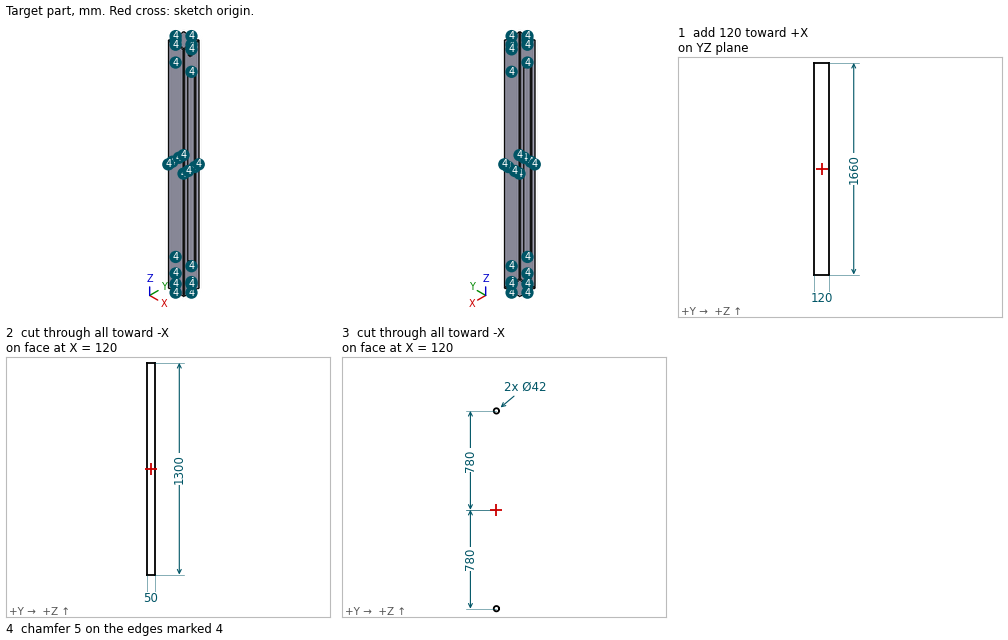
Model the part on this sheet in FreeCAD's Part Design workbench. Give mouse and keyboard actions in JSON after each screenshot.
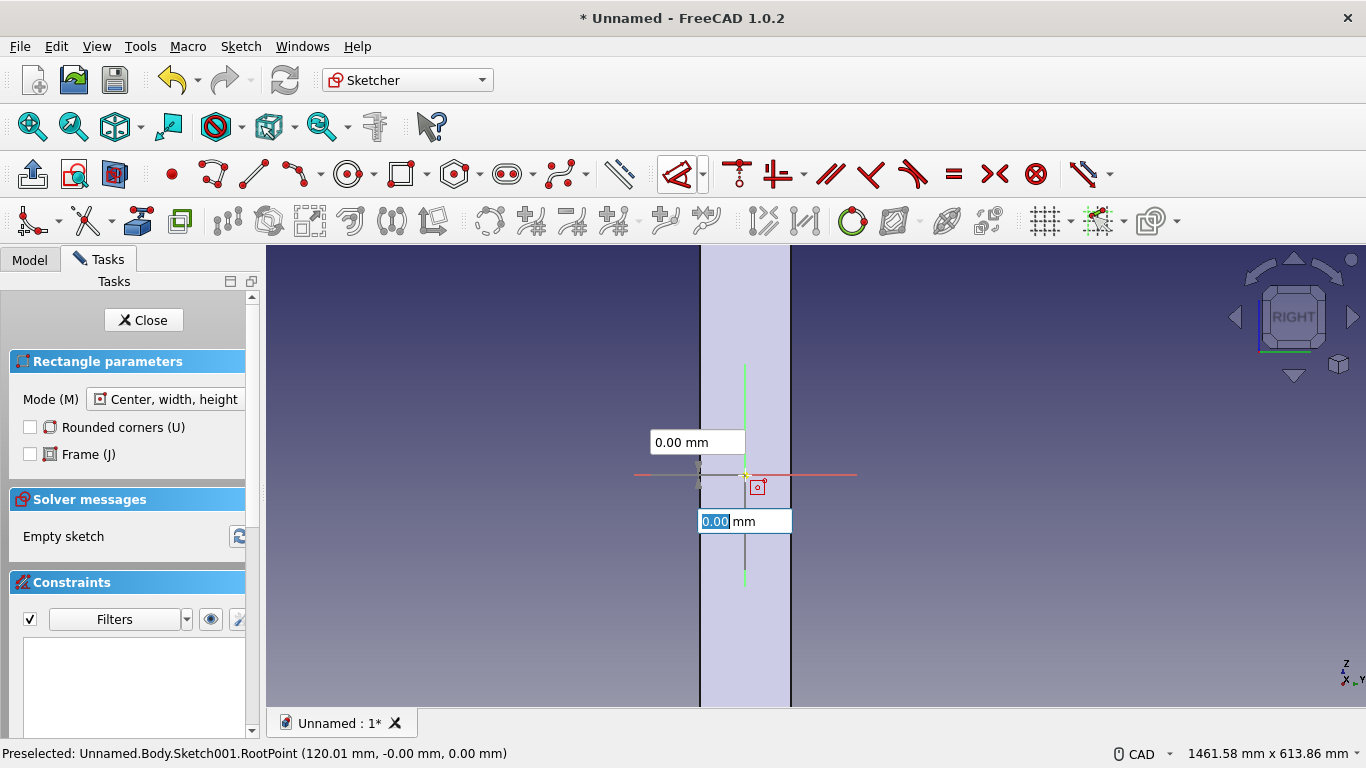
{"action": "scroll", "coordinate": [748, 476], "scroll_direction": "down", "scroll_amount": 6}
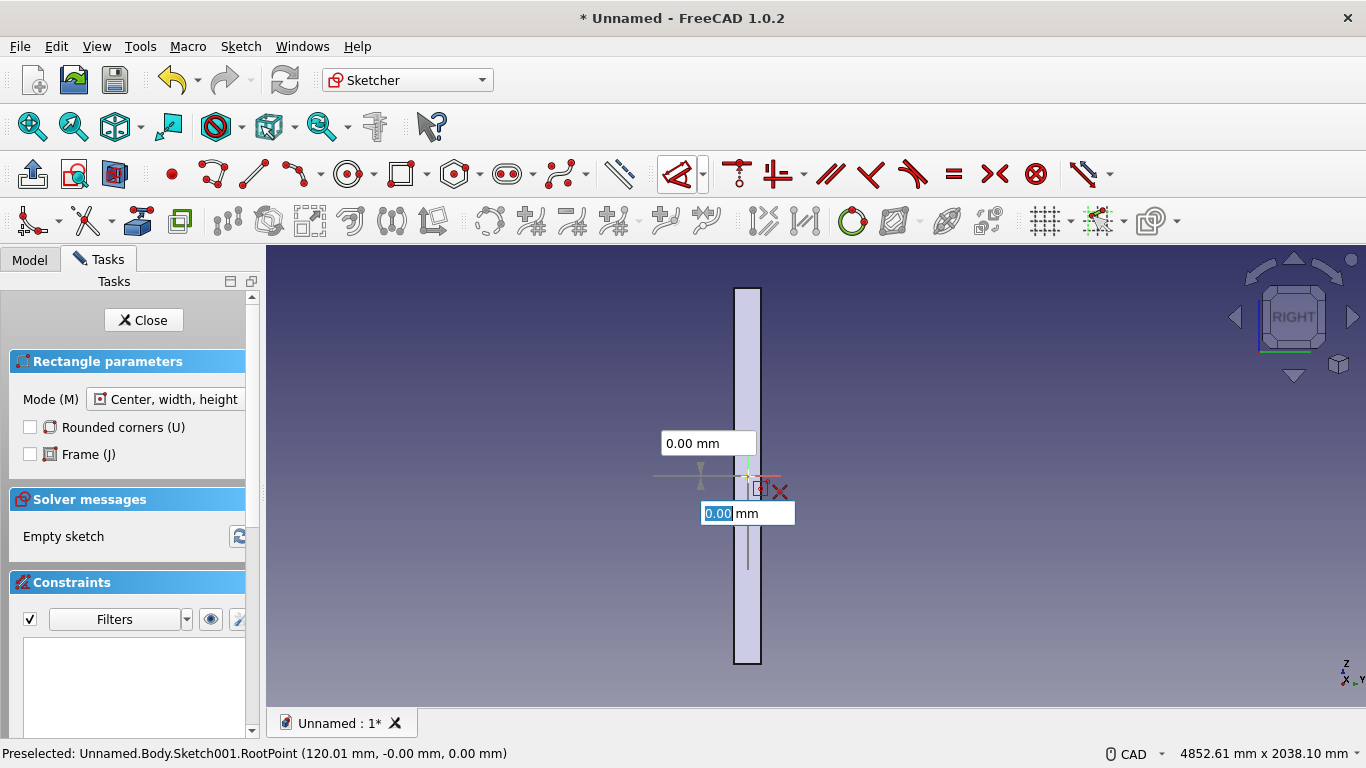
{"action": "scroll", "coordinate": [753, 329], "scroll_direction": "up", "scroll_amount": 6}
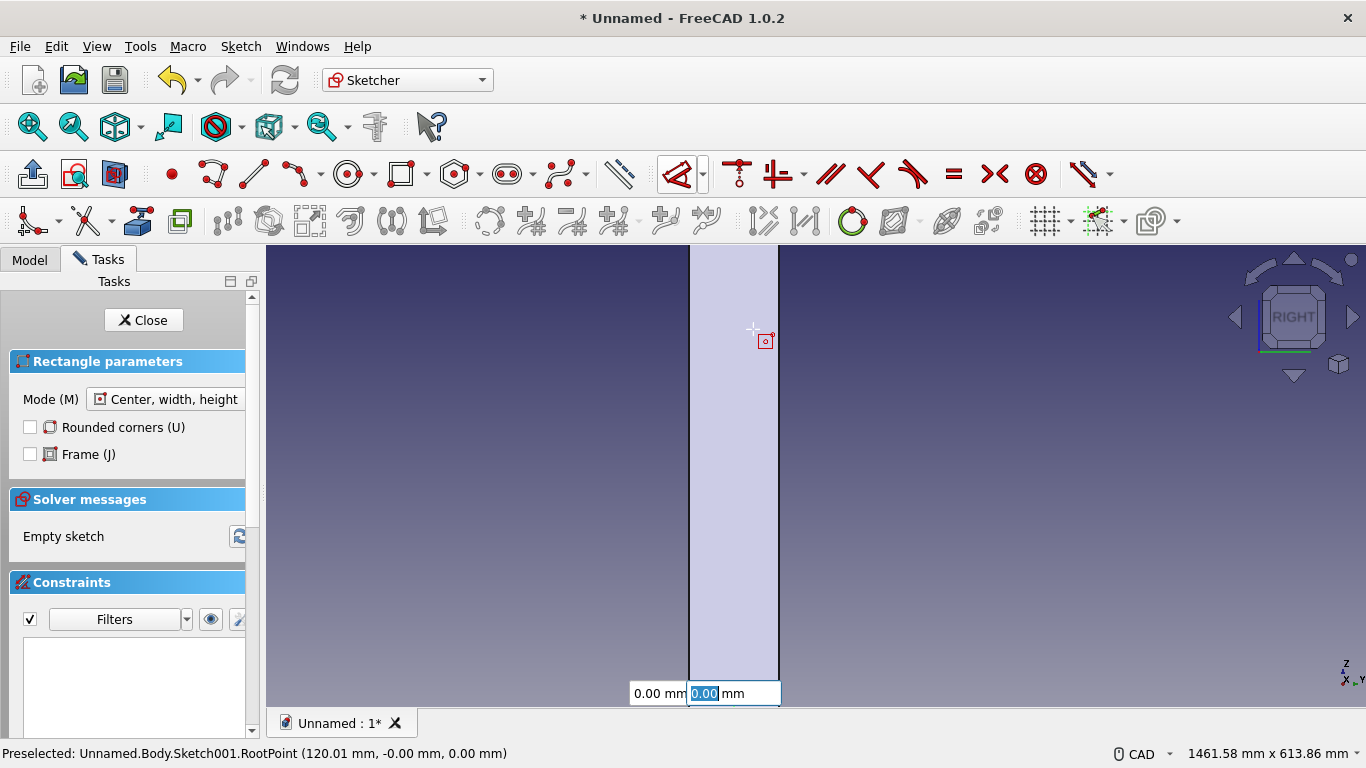
{"action": "left_click", "coordinate": [753, 328]}
{"action": "key", "text": "Escape"}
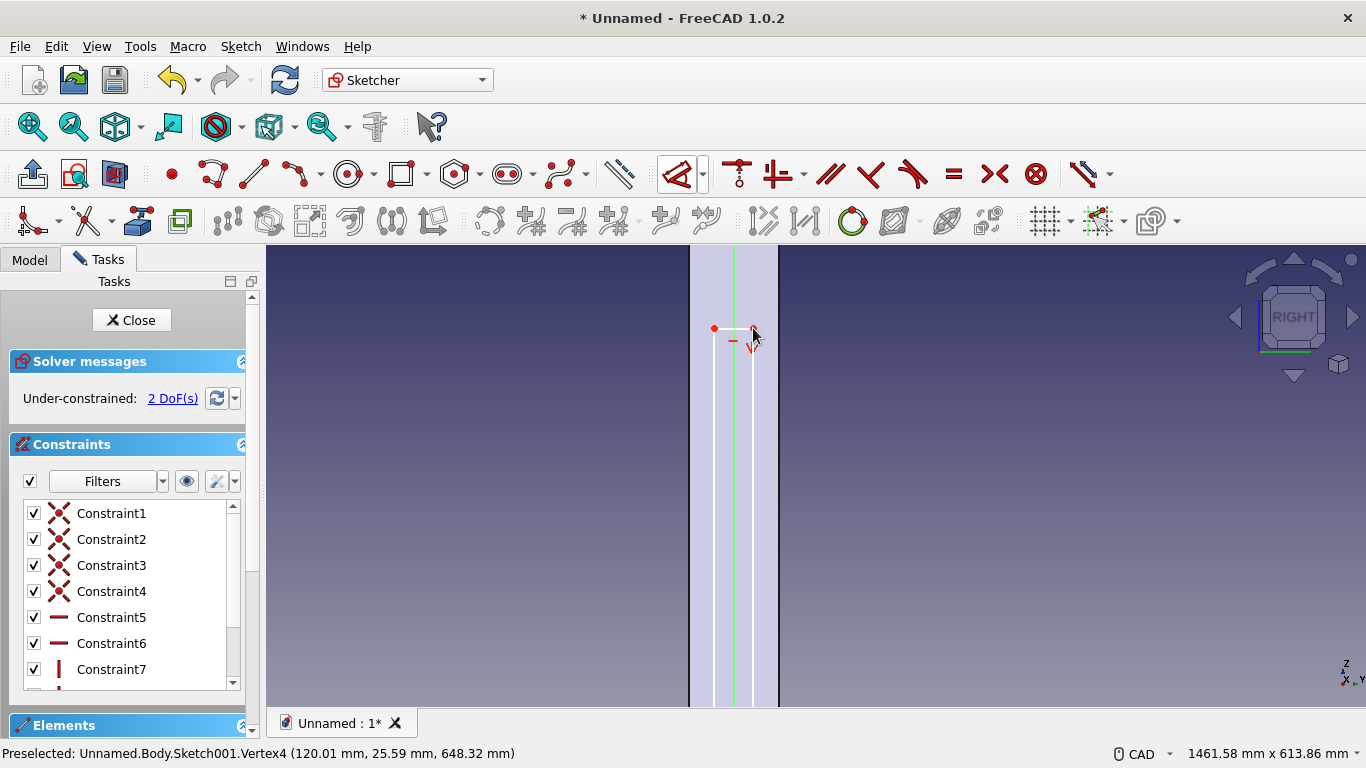
{"action": "key", "text": "d"}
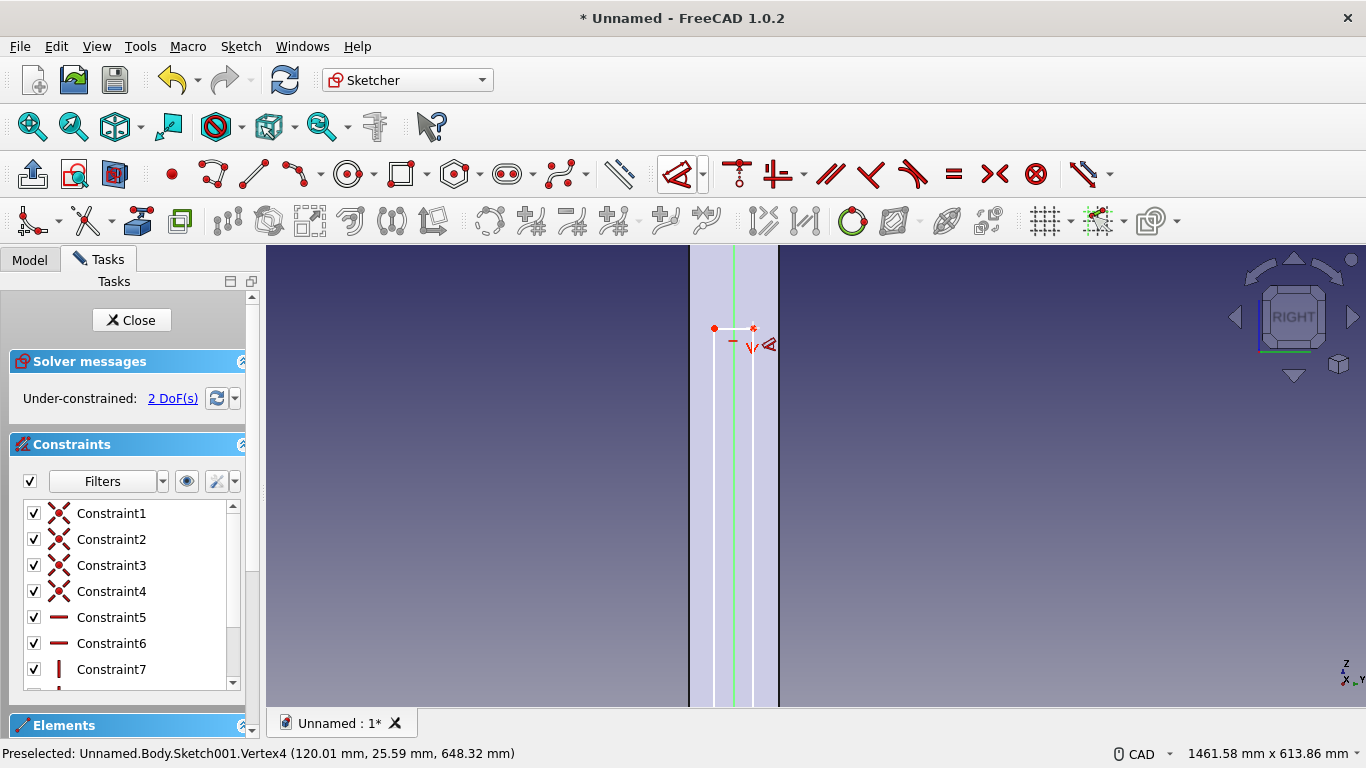
{"action": "scroll", "coordinate": [753, 329], "scroll_direction": "down", "scroll_amount": 6}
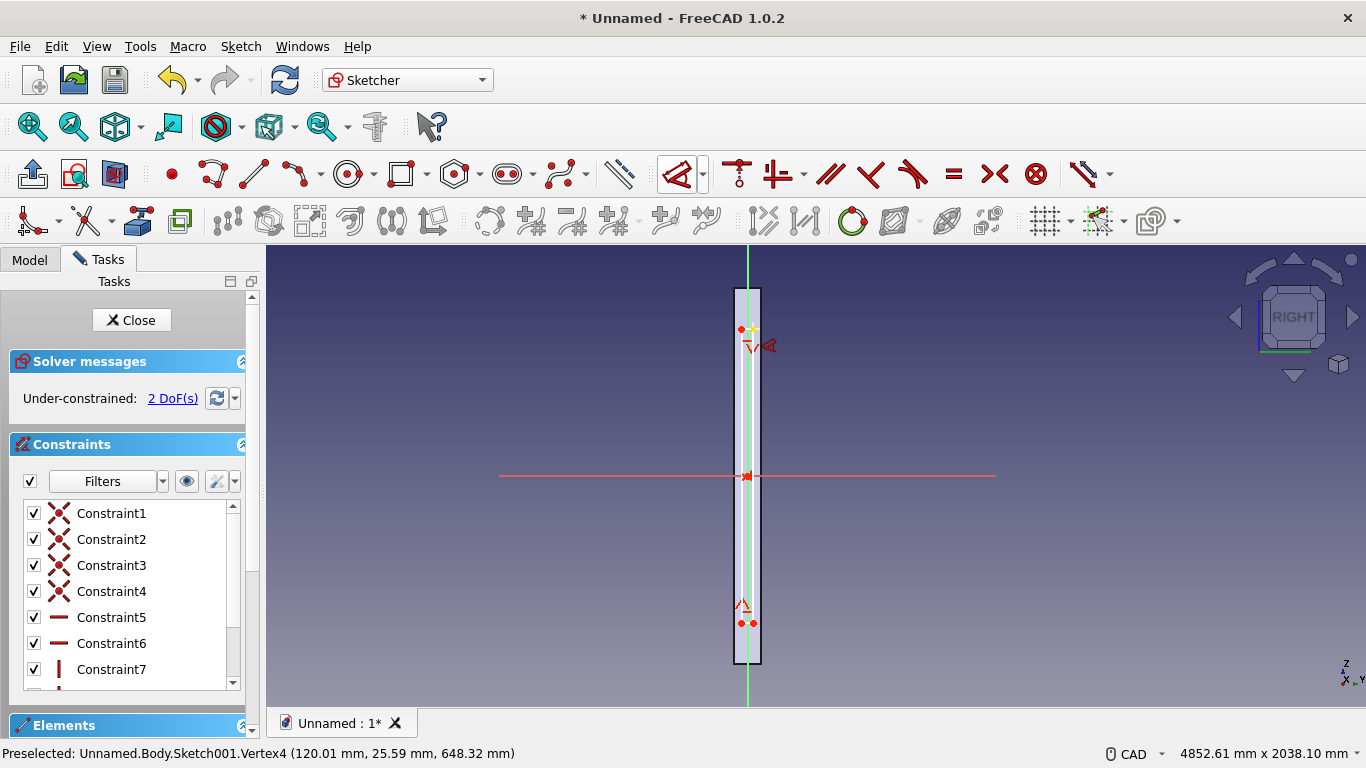
{"action": "scroll", "coordinate": [746, 623], "scroll_direction": "up", "scroll_amount": 7}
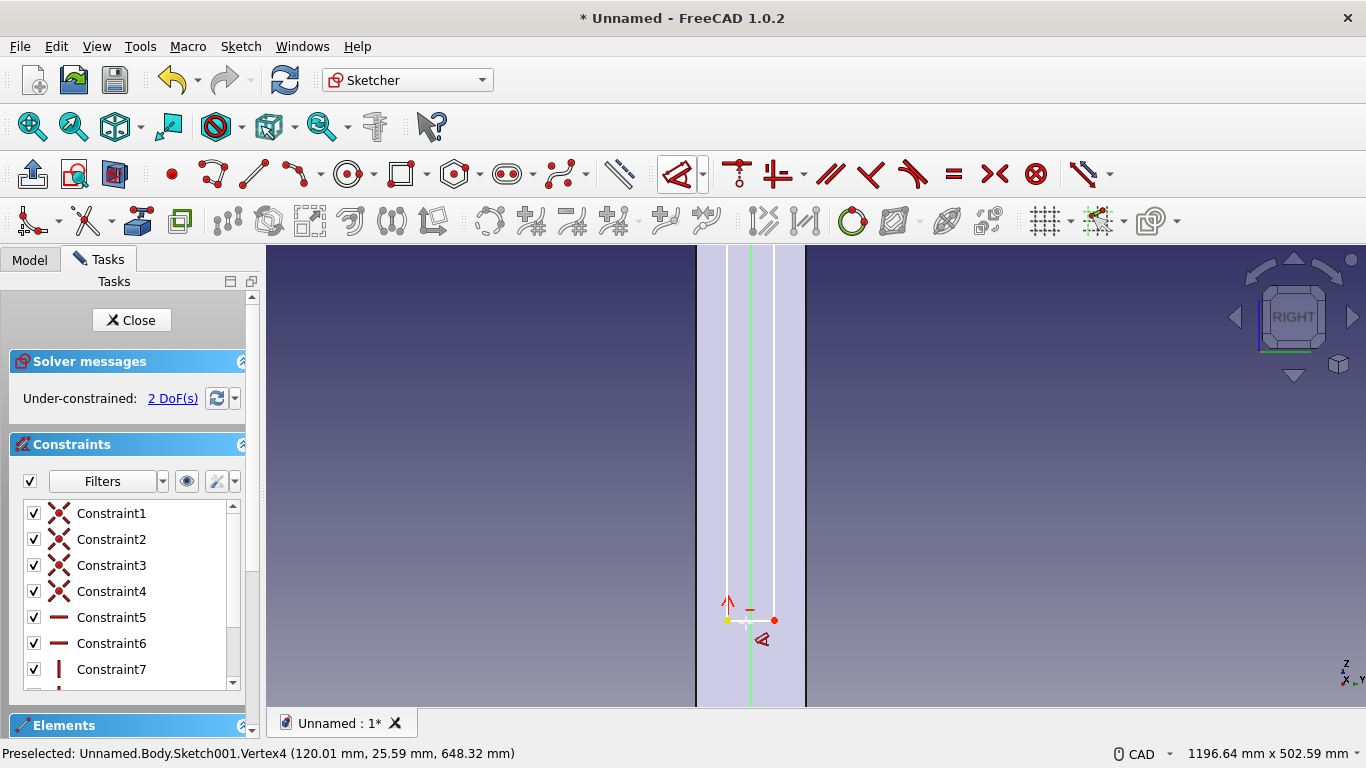
{"action": "left_click", "coordinate": [746, 621]}
{"action": "left_click", "coordinate": [734, 655]}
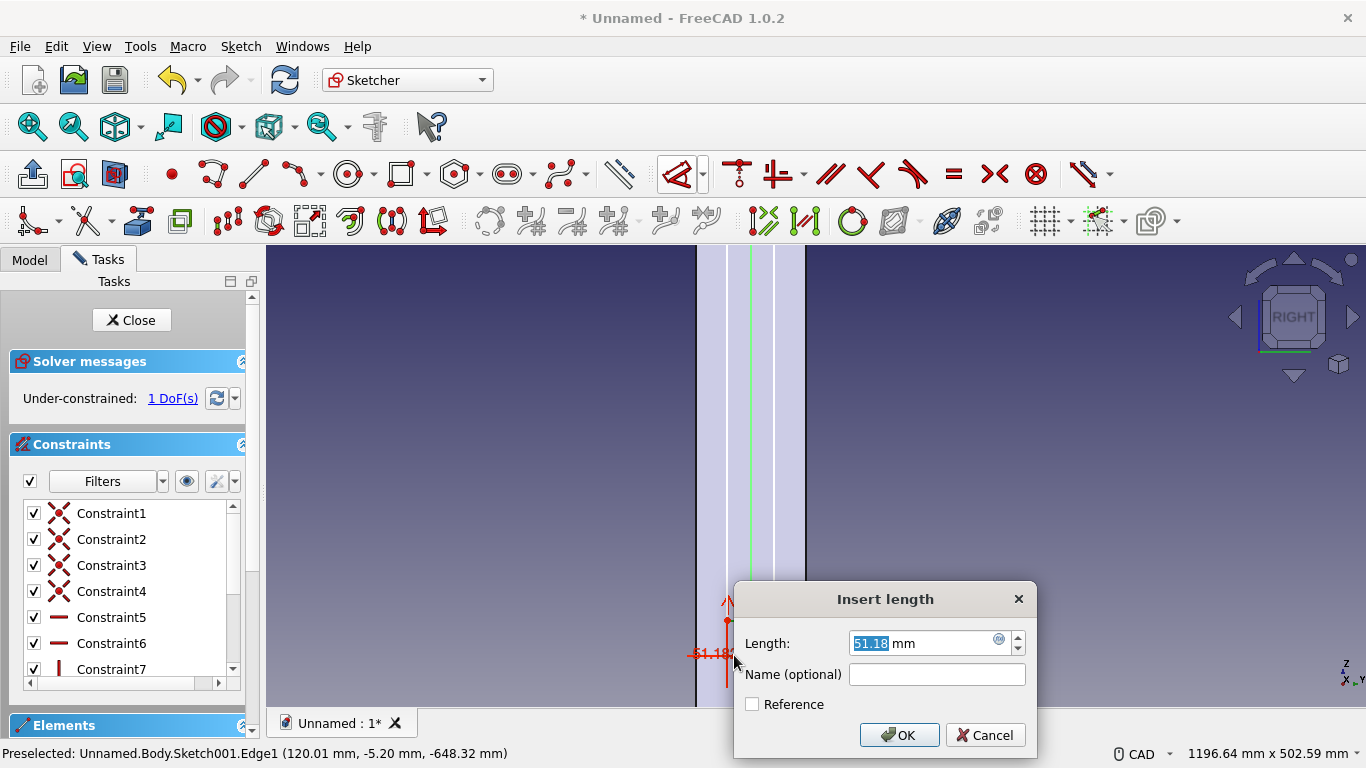
{"action": "type", "text": "50"}
{"action": "key", "text": "Return"}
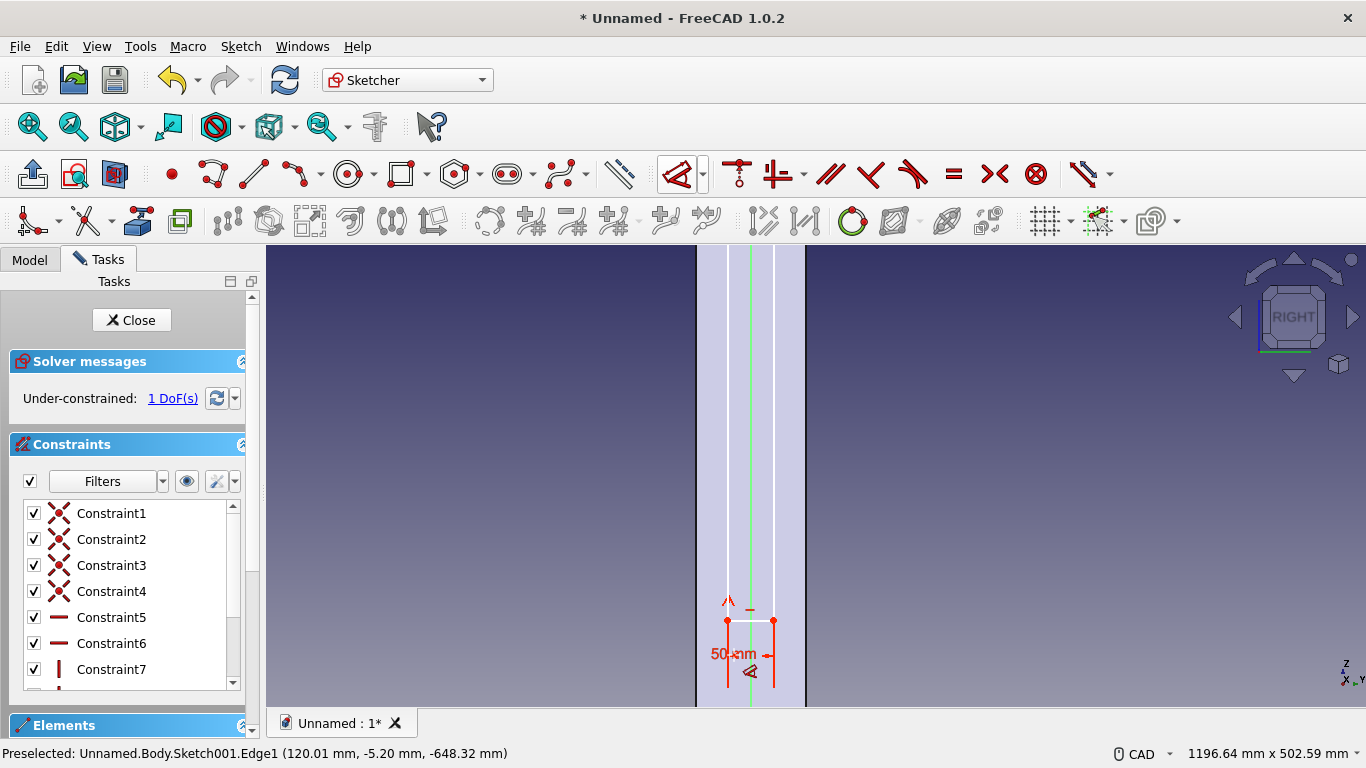
{"action": "left_click", "coordinate": [774, 382]}
{"action": "left_click", "coordinate": [808, 447]}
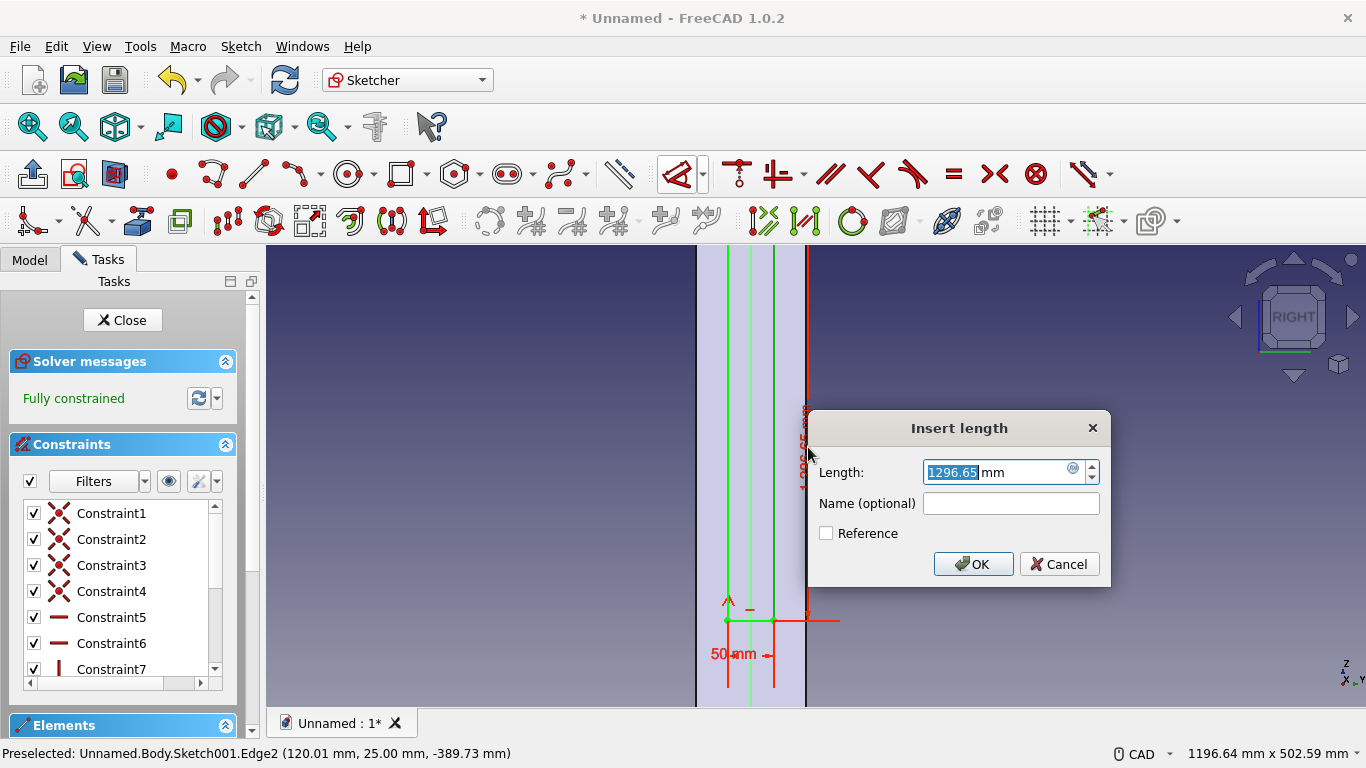
{"action": "type", "text": "1300"}
{"action": "key", "text": "Return"}
{"action": "key", "text": "Escape"}